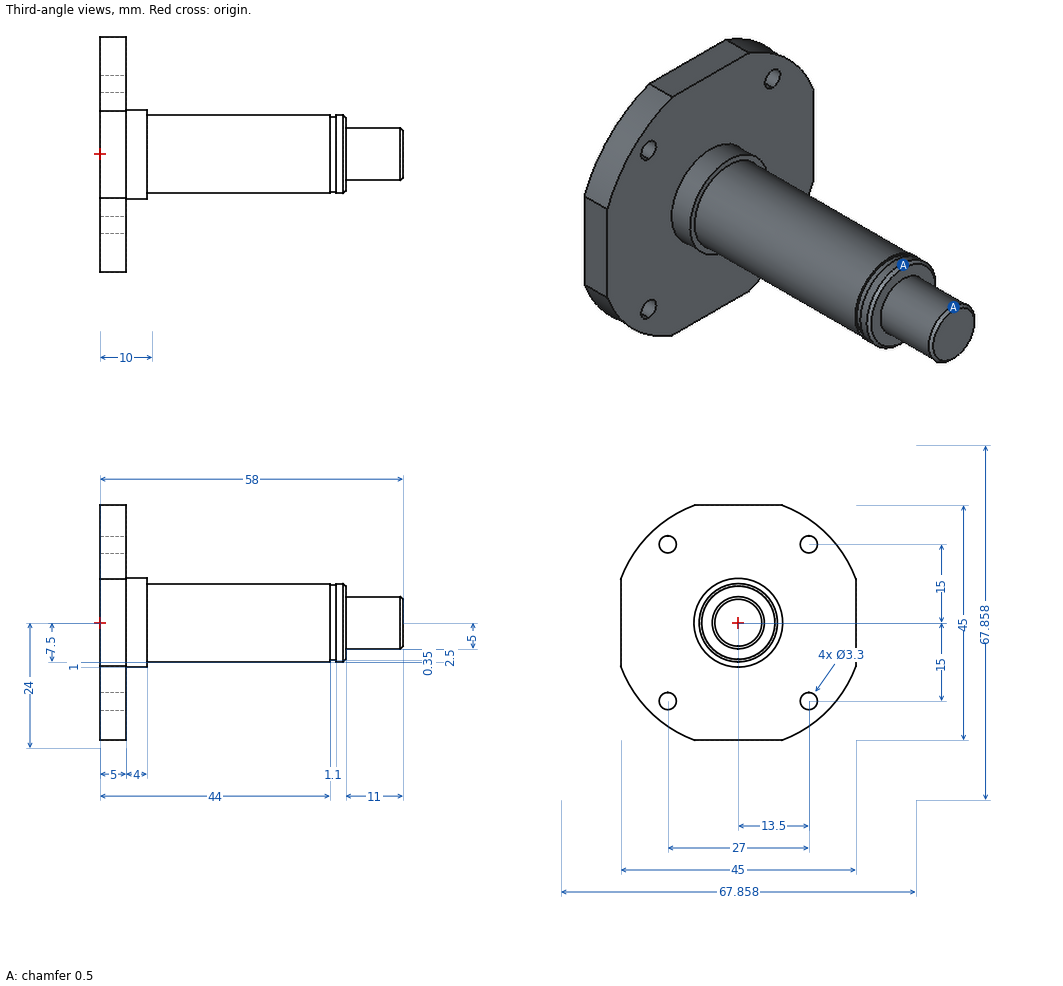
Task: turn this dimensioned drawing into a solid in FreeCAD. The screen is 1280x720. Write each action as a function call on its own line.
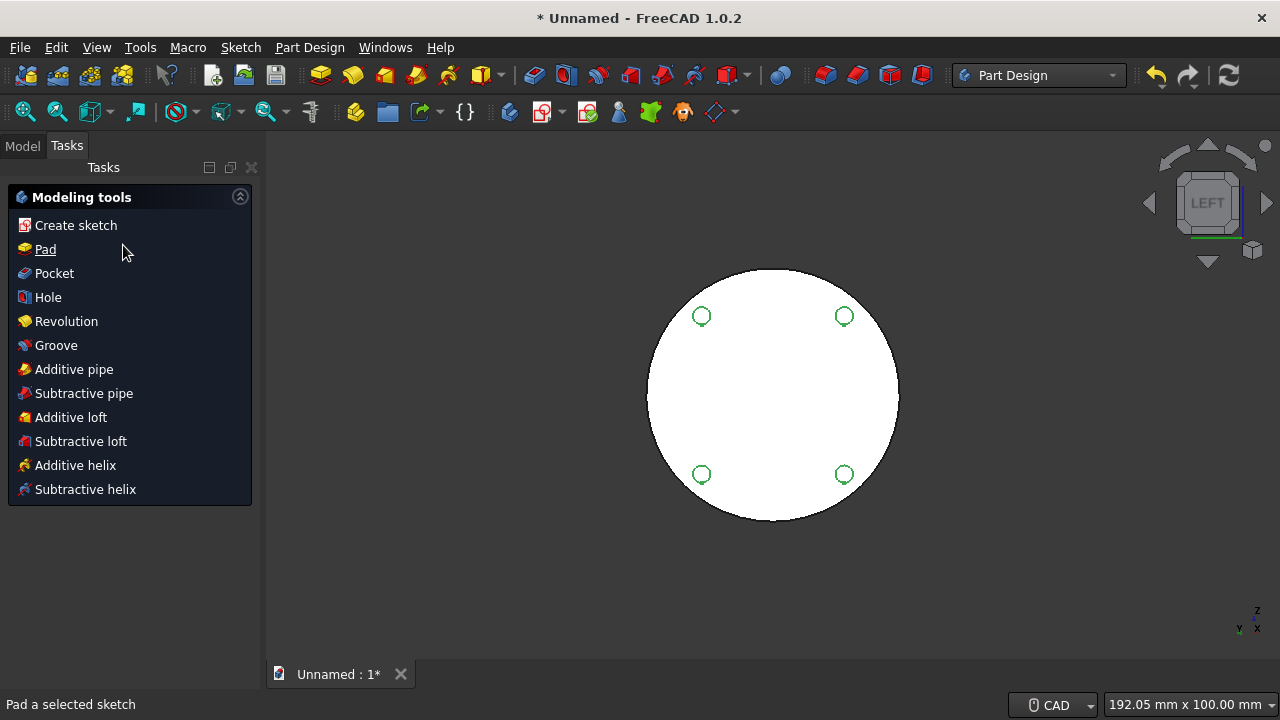
click(536, 76)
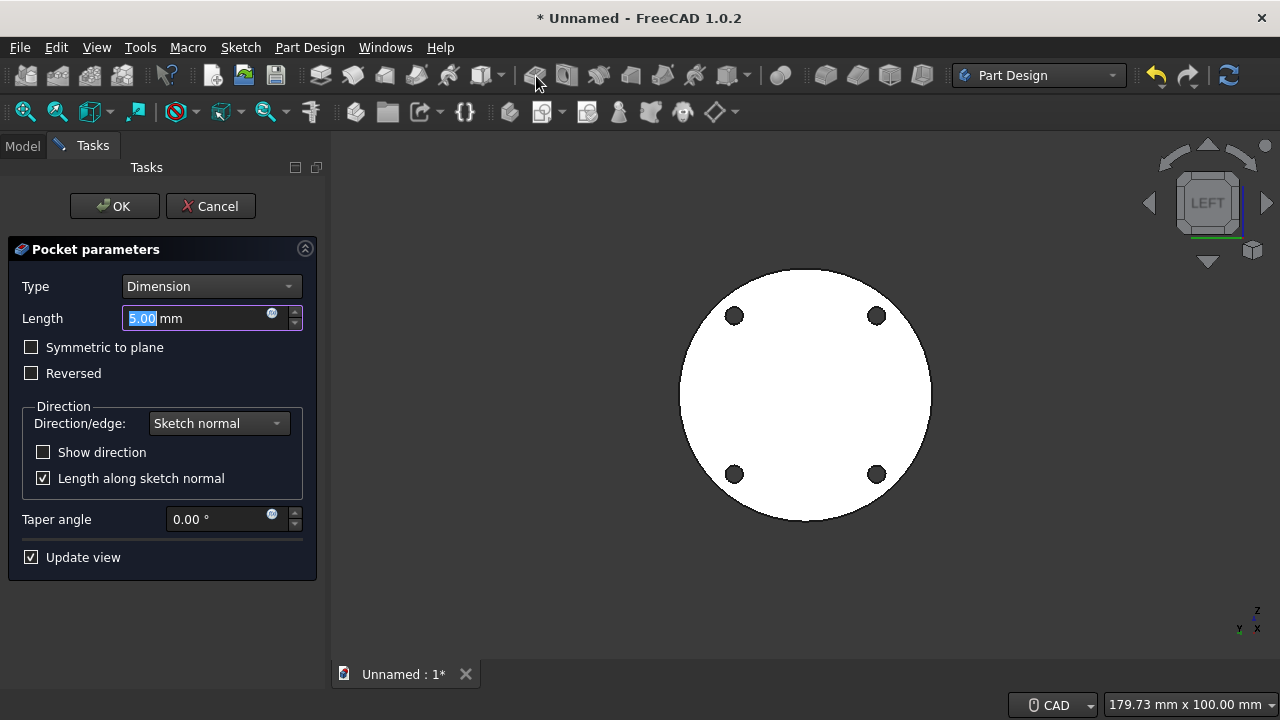
click(212, 286)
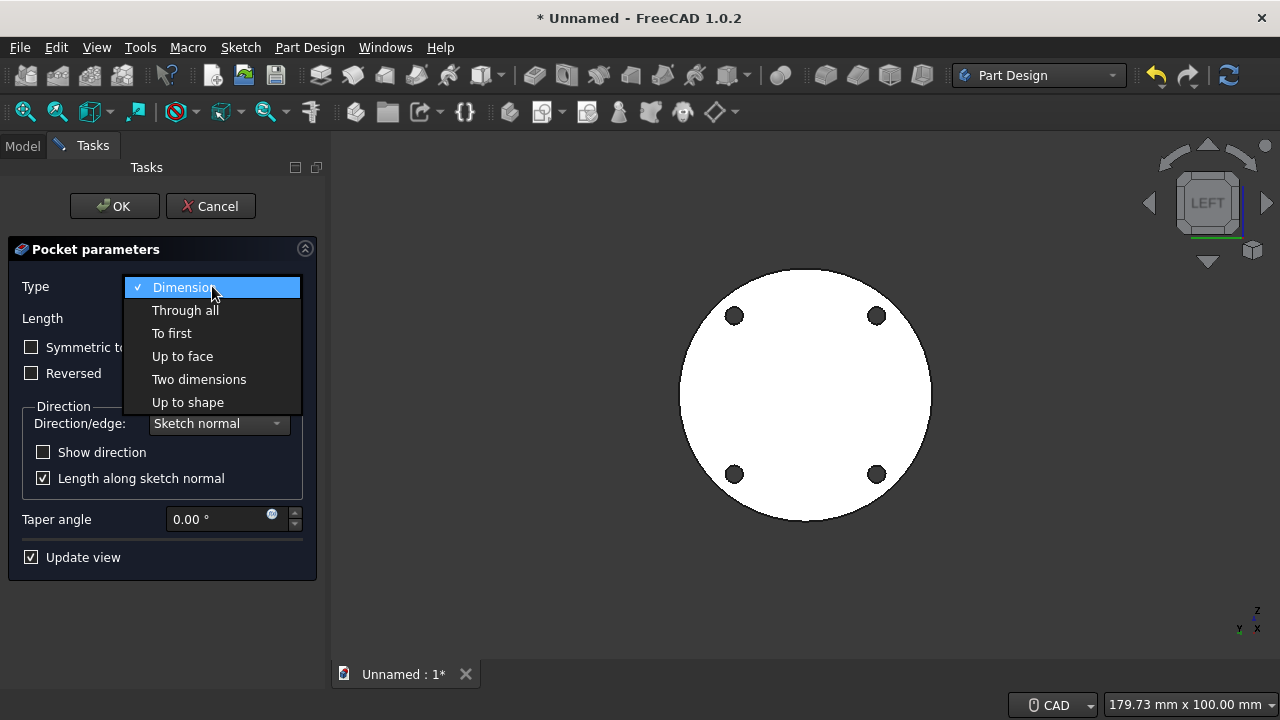
click(212, 310)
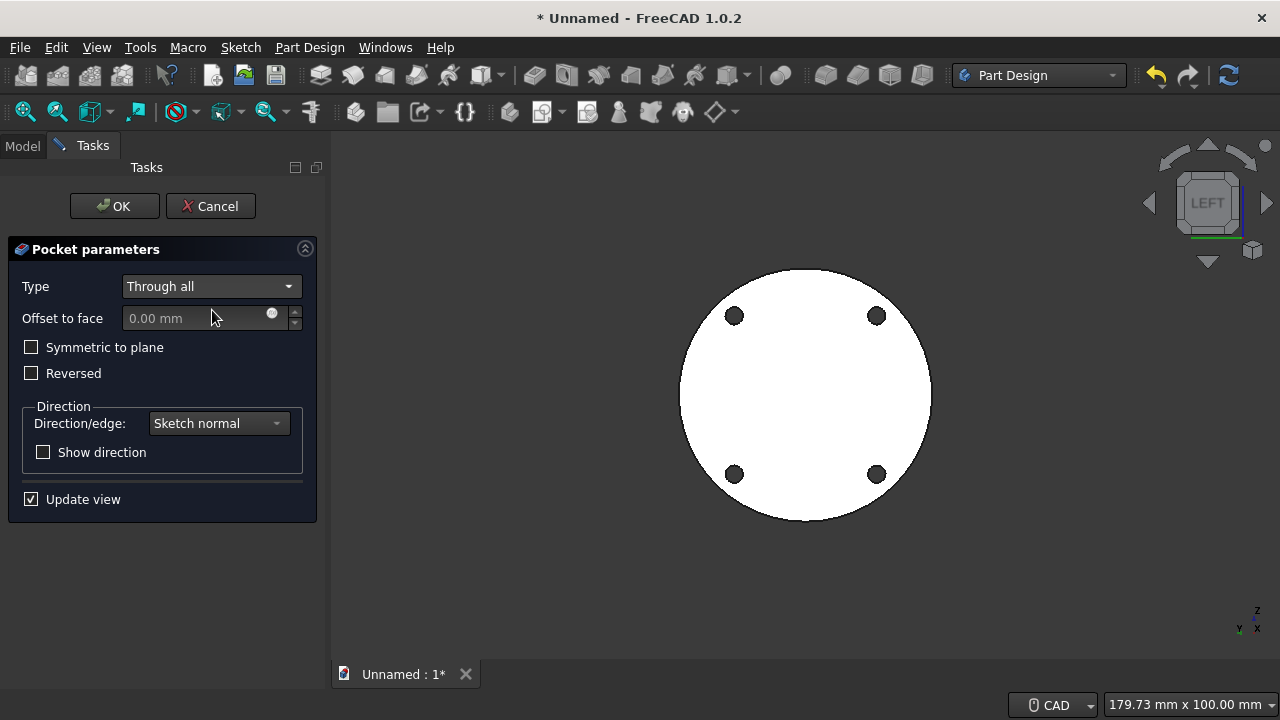
click(115, 206)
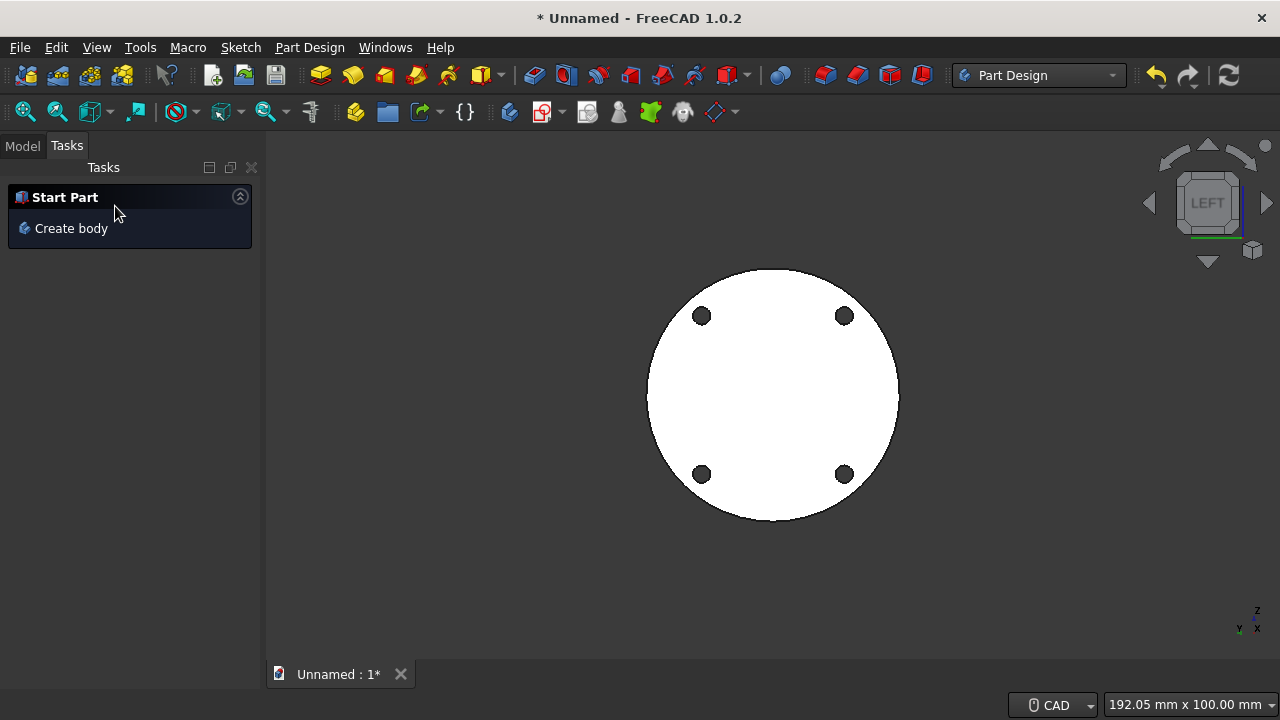
click(773, 394)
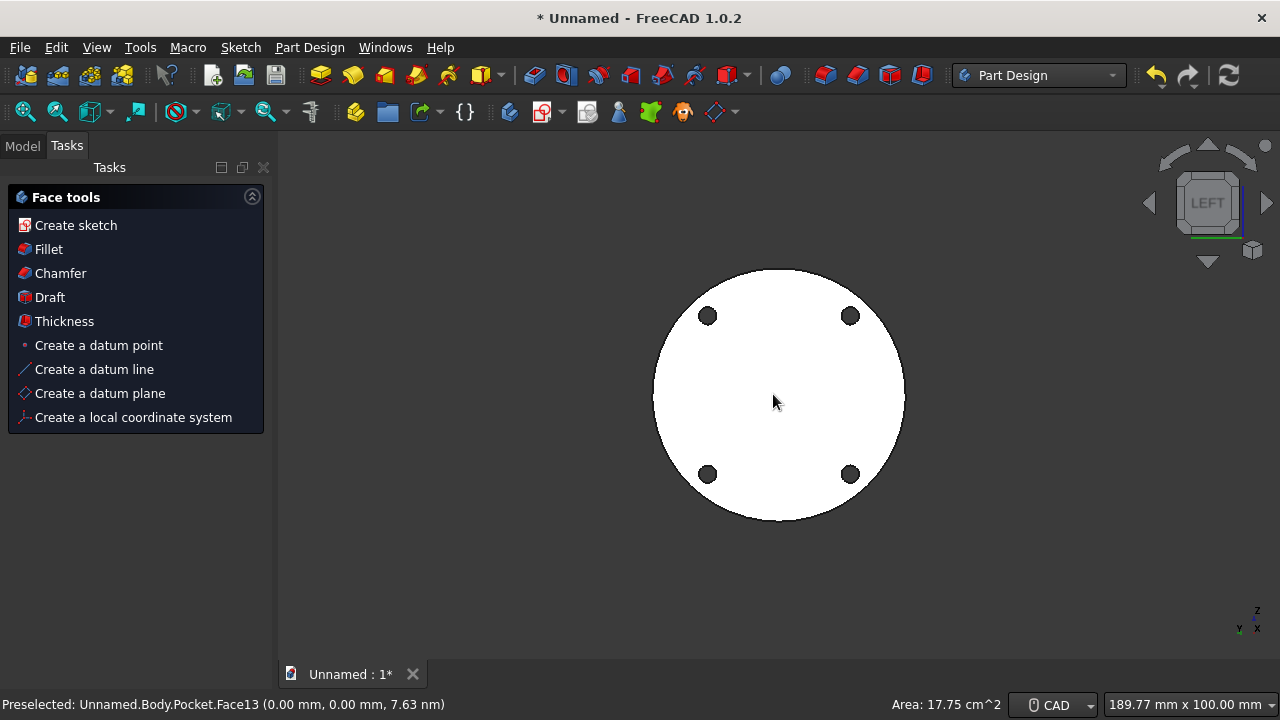
click(542, 112)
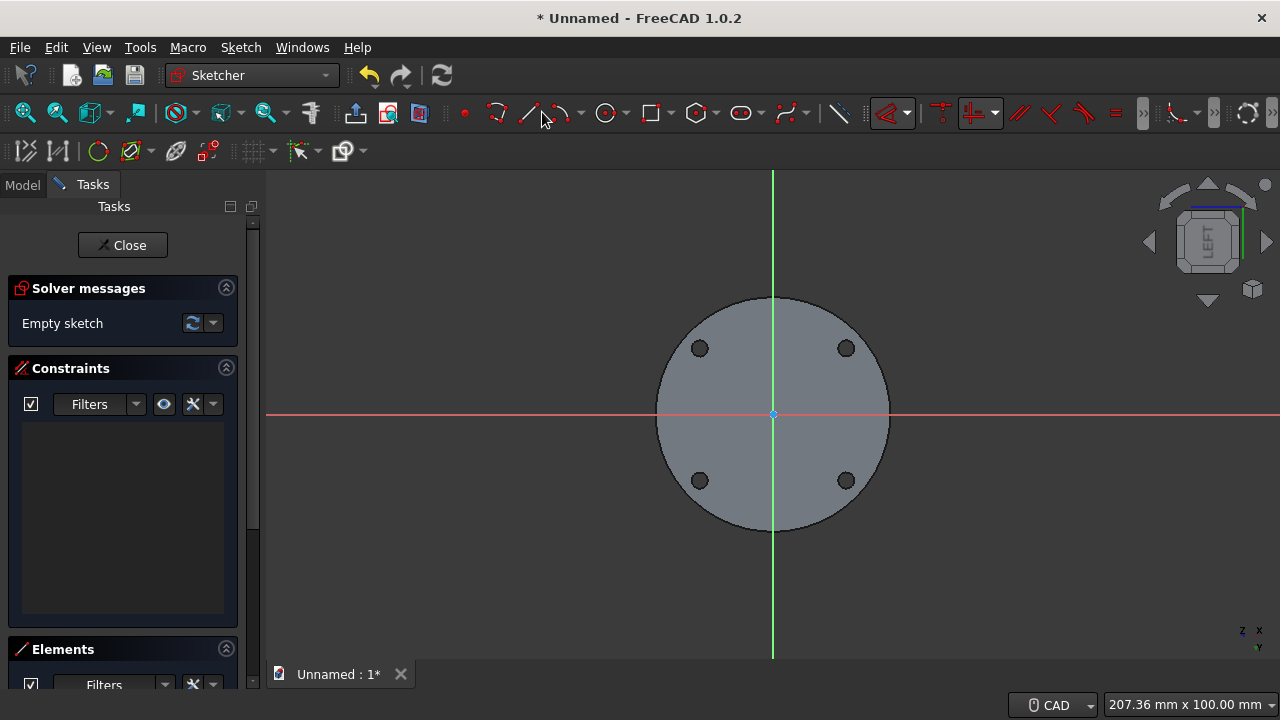
key(g)
key(v)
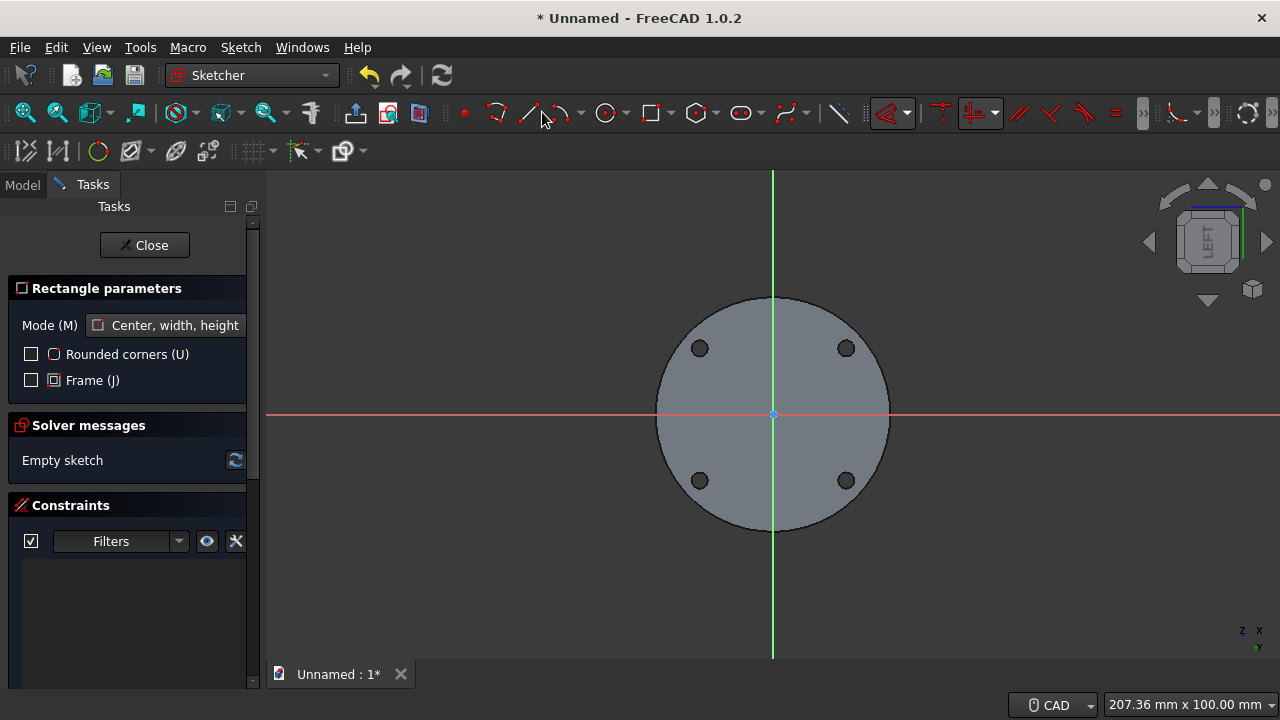
click(773, 414)
click(939, 249)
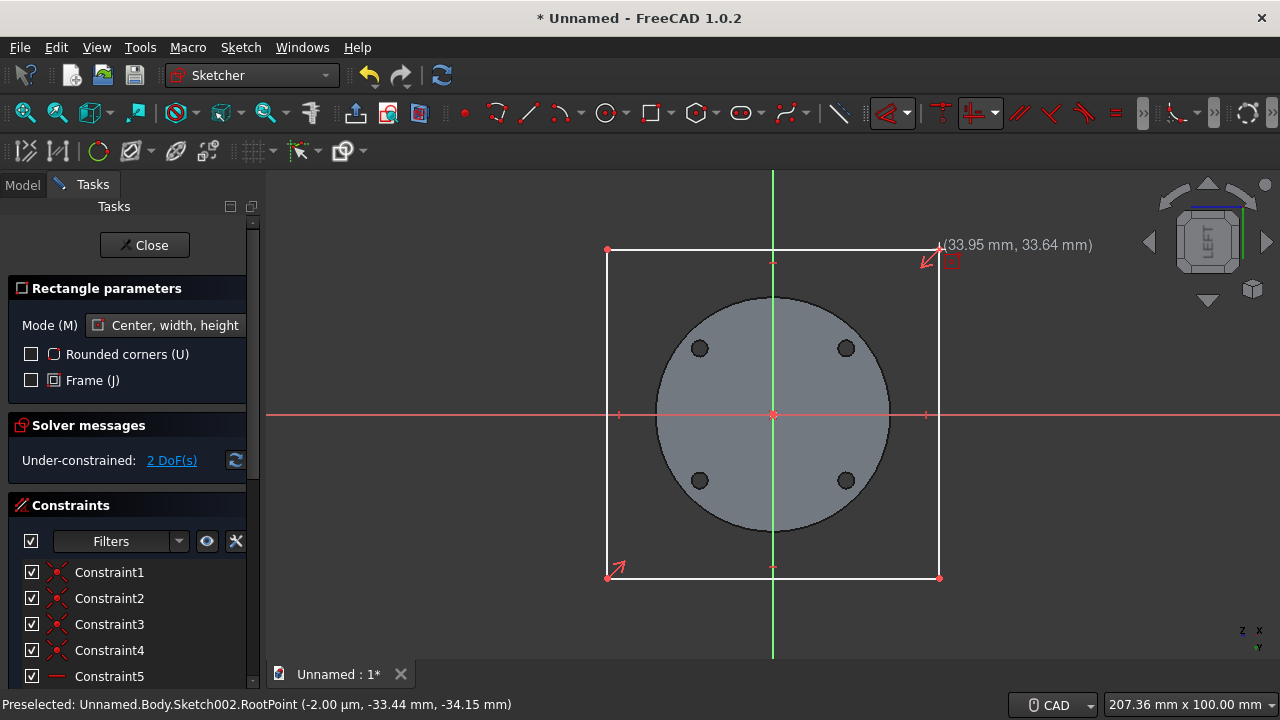
click(773, 414)
click(883, 304)
key(Escape)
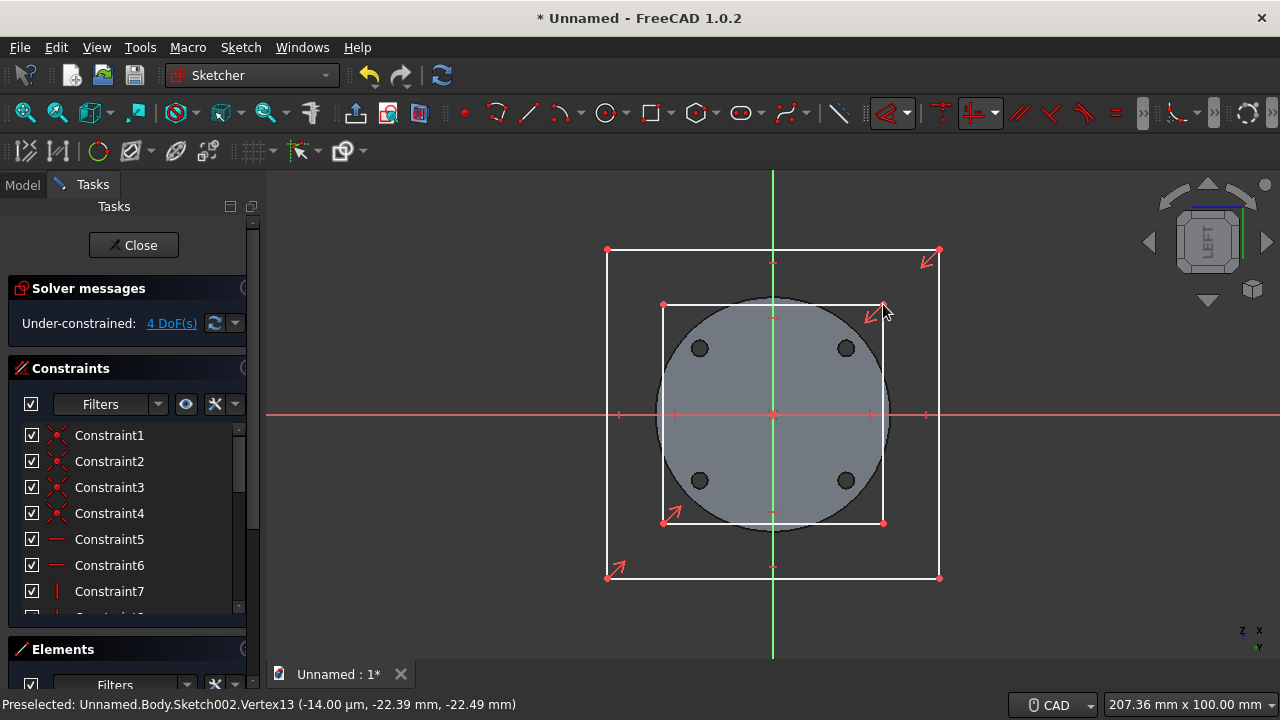
click(729, 524)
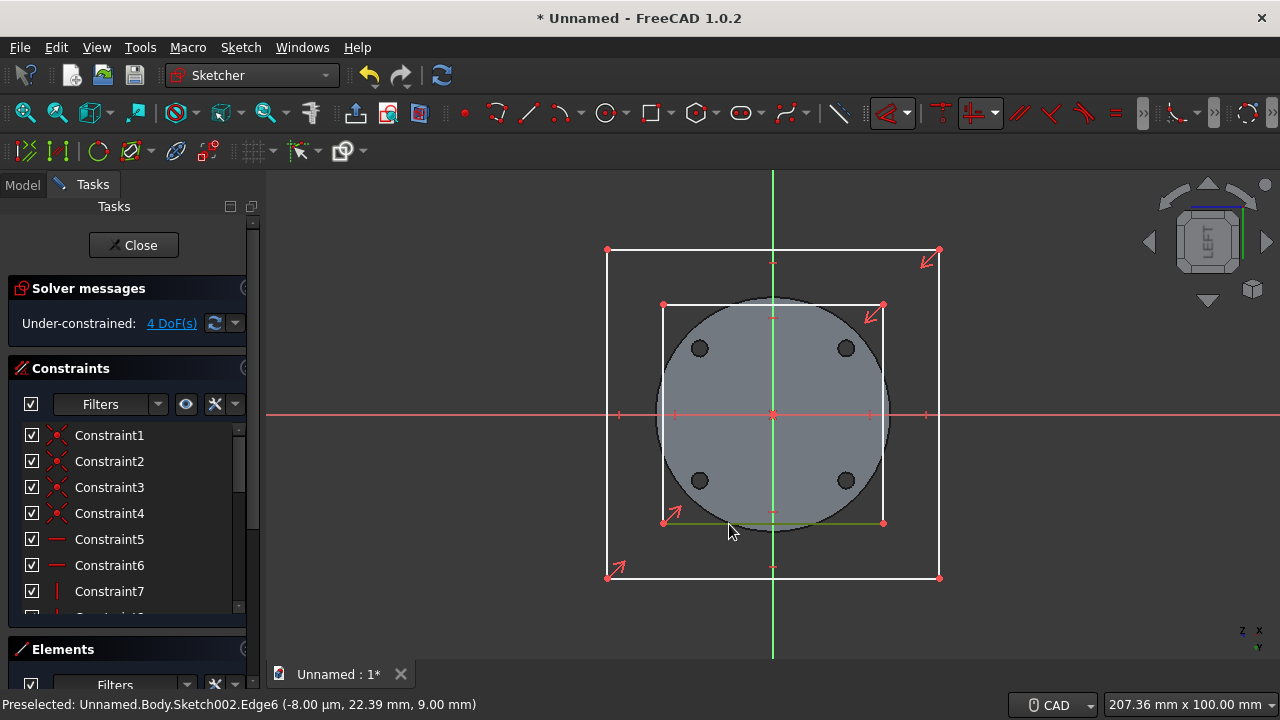
click(910, 114)